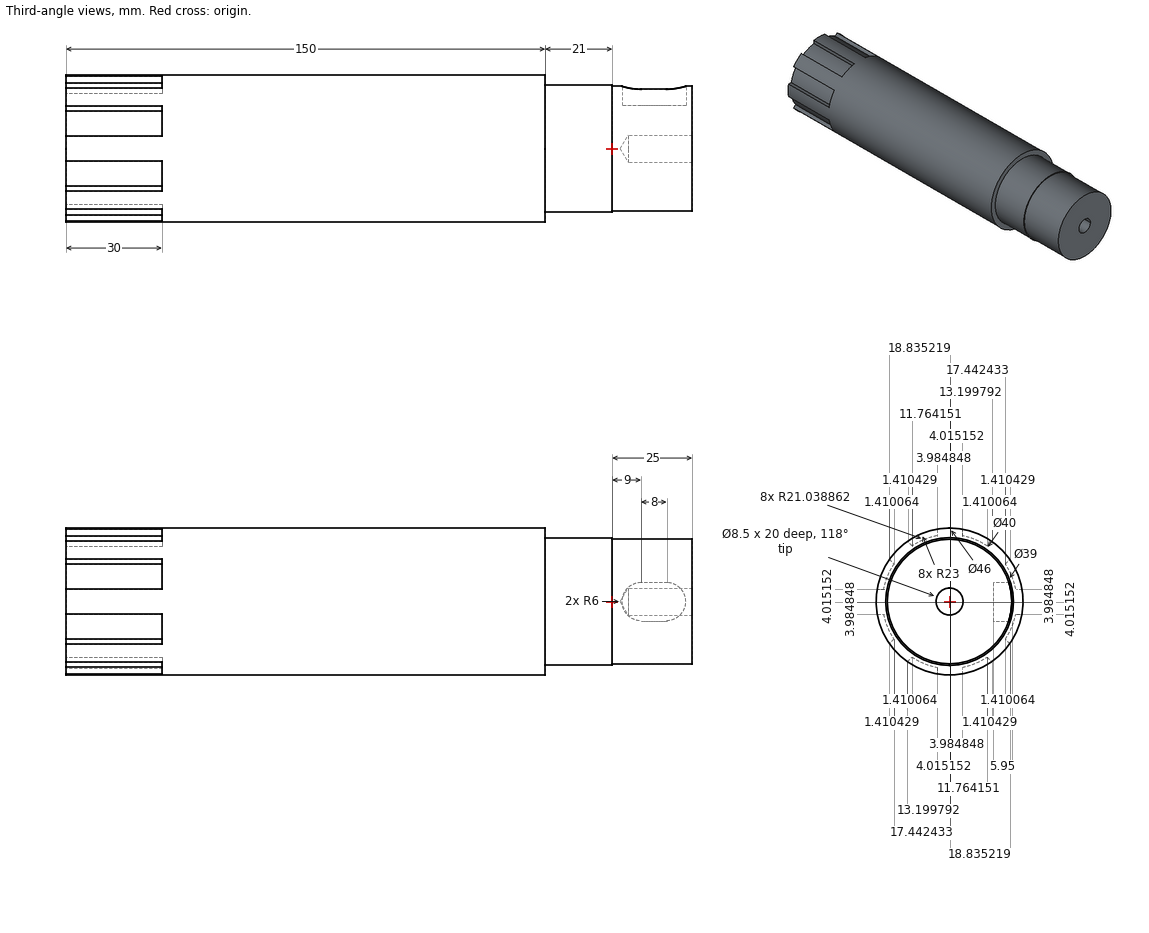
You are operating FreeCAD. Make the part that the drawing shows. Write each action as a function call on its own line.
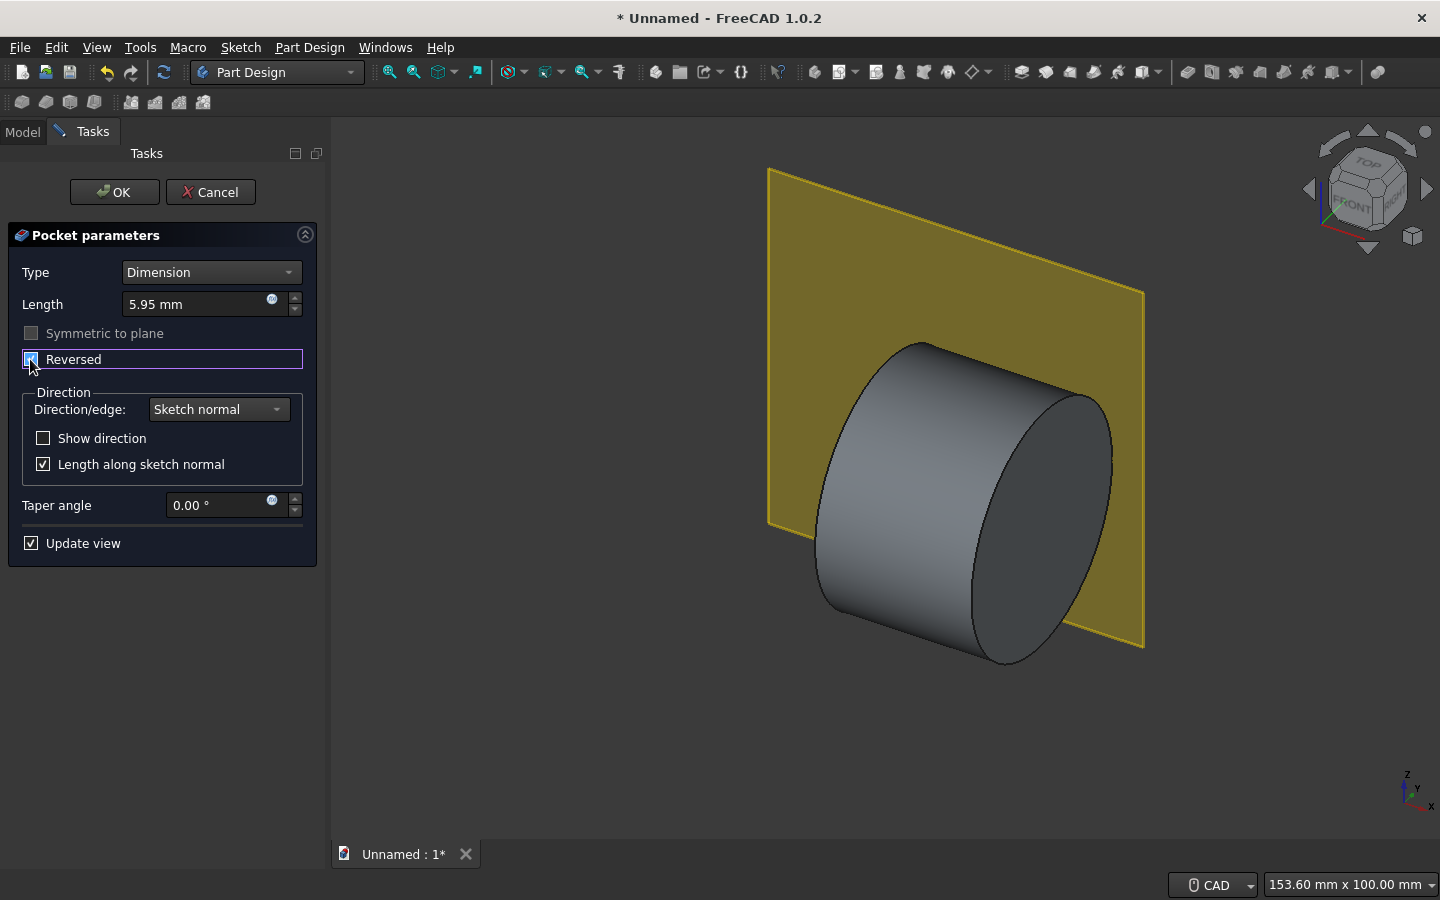
click(115, 192)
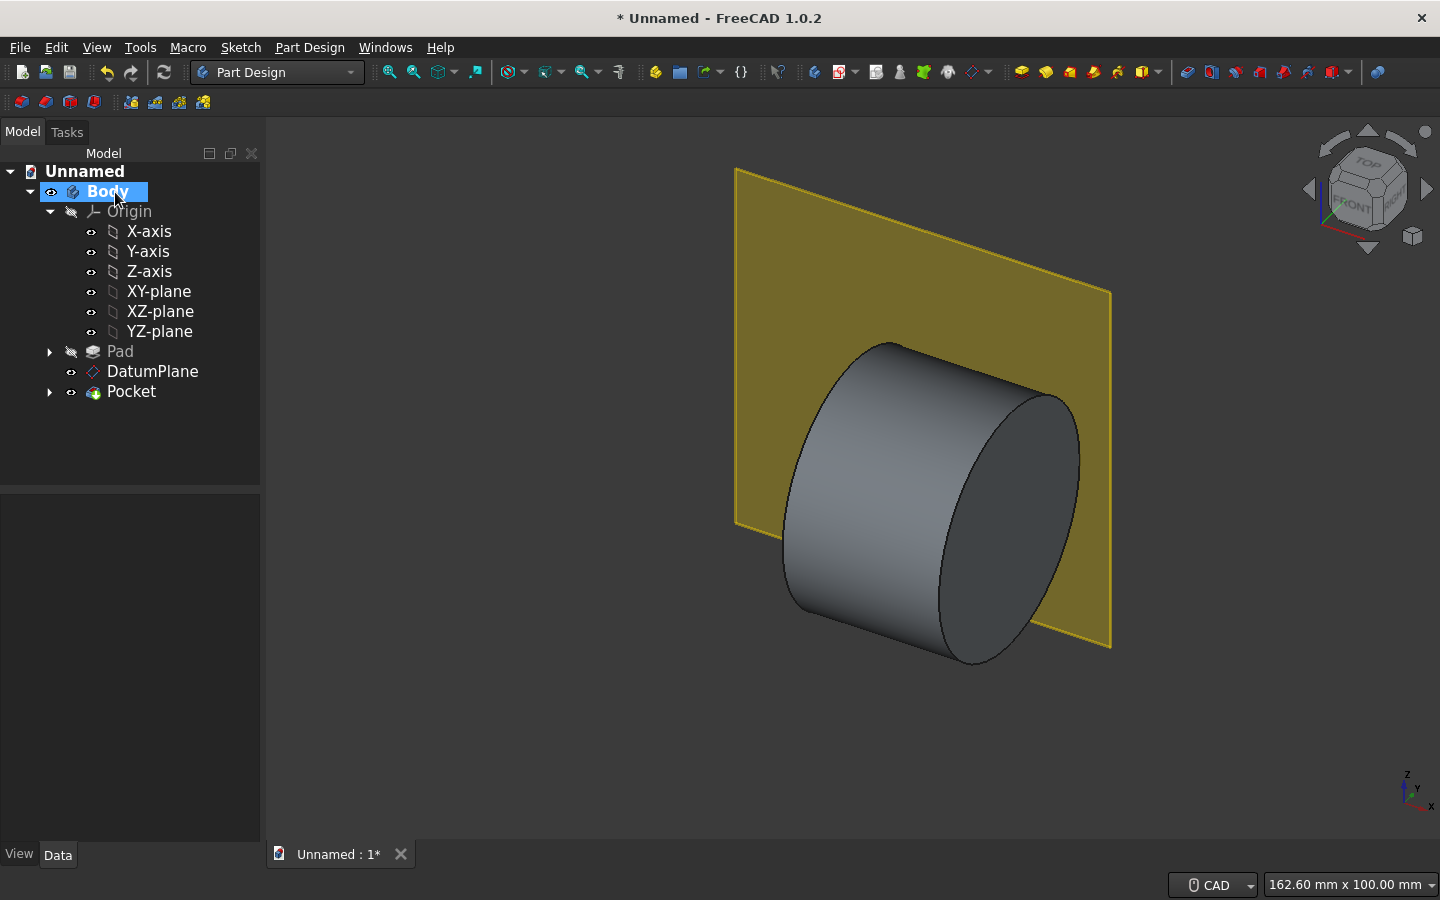
click(116, 372)
key(space)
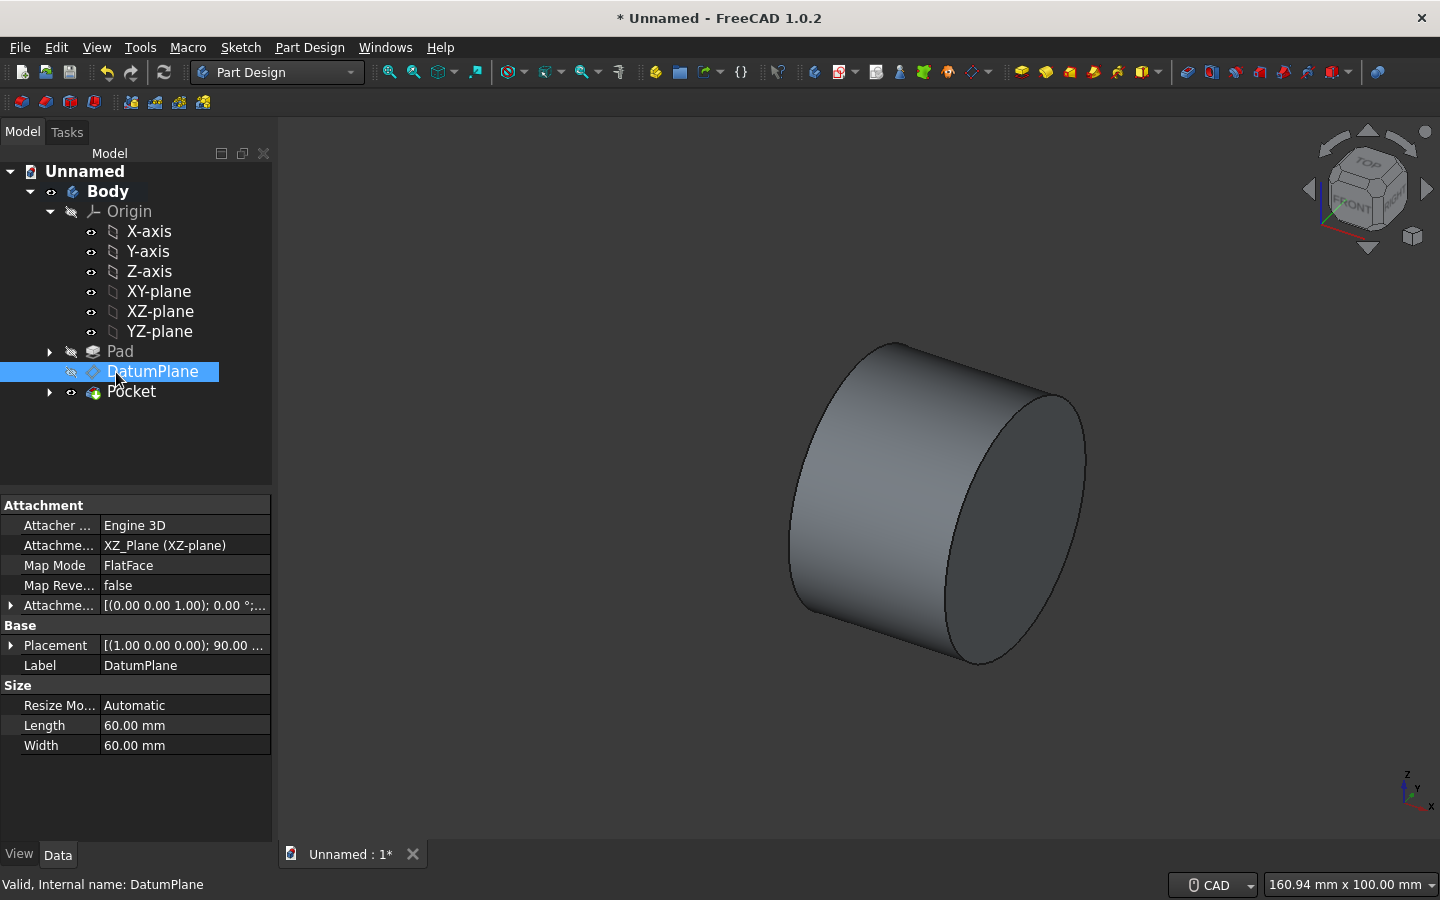
click(318, 799)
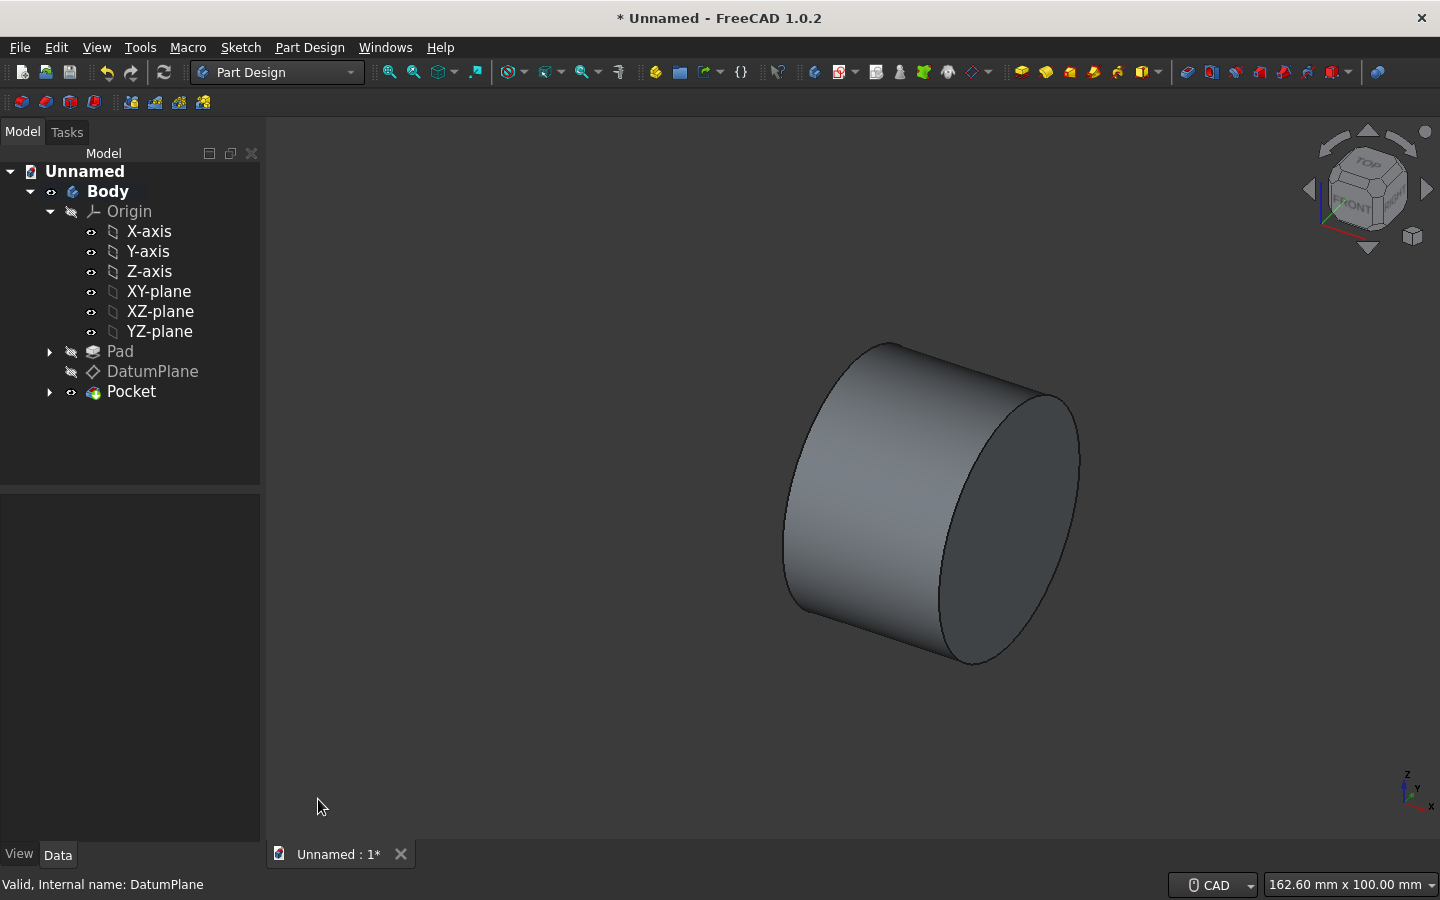
click(840, 72)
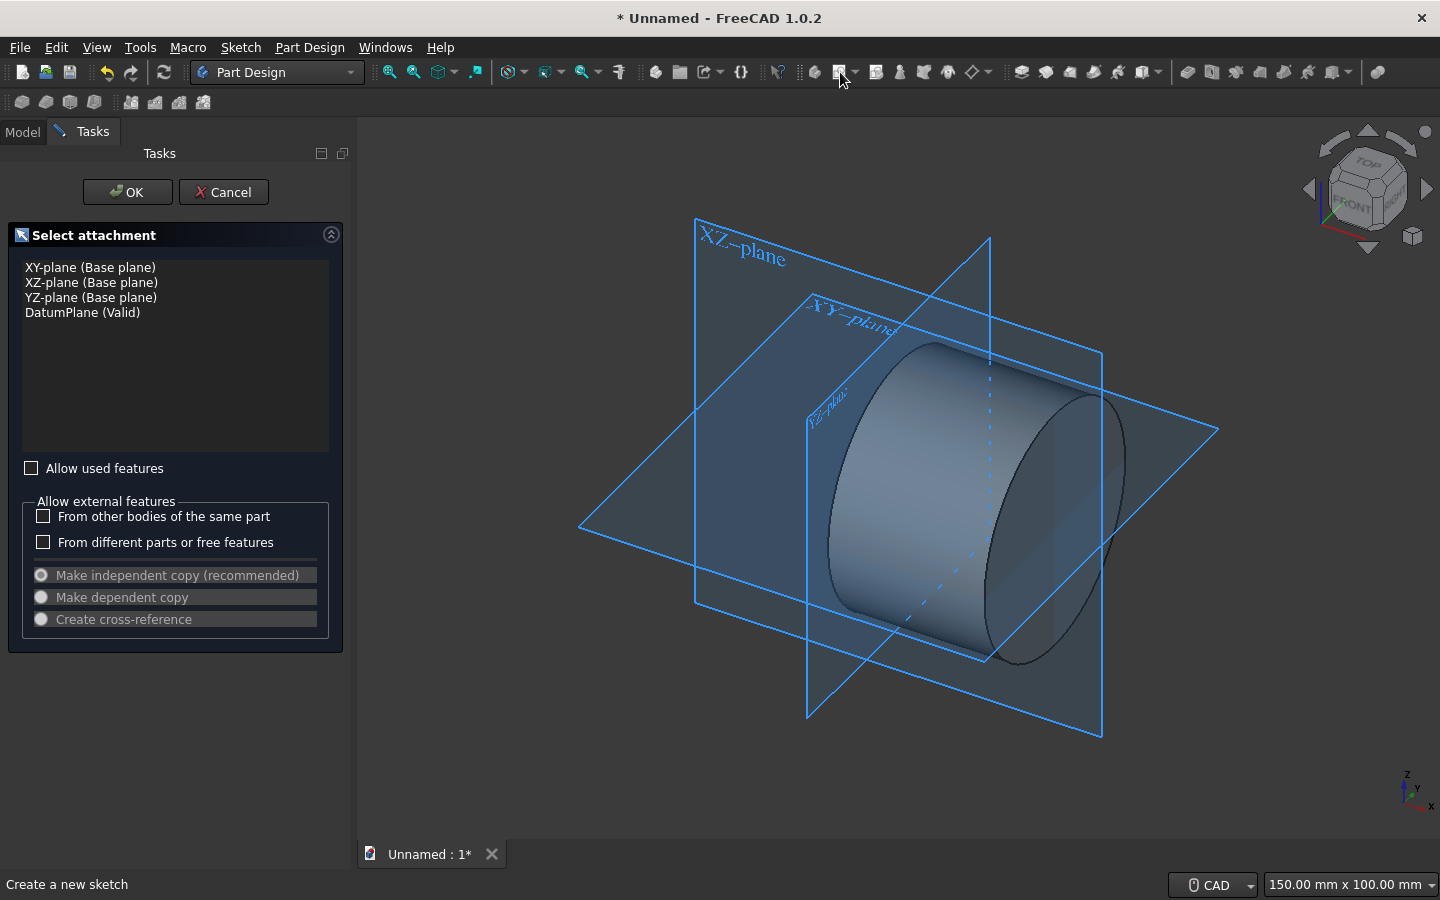
click(82, 298)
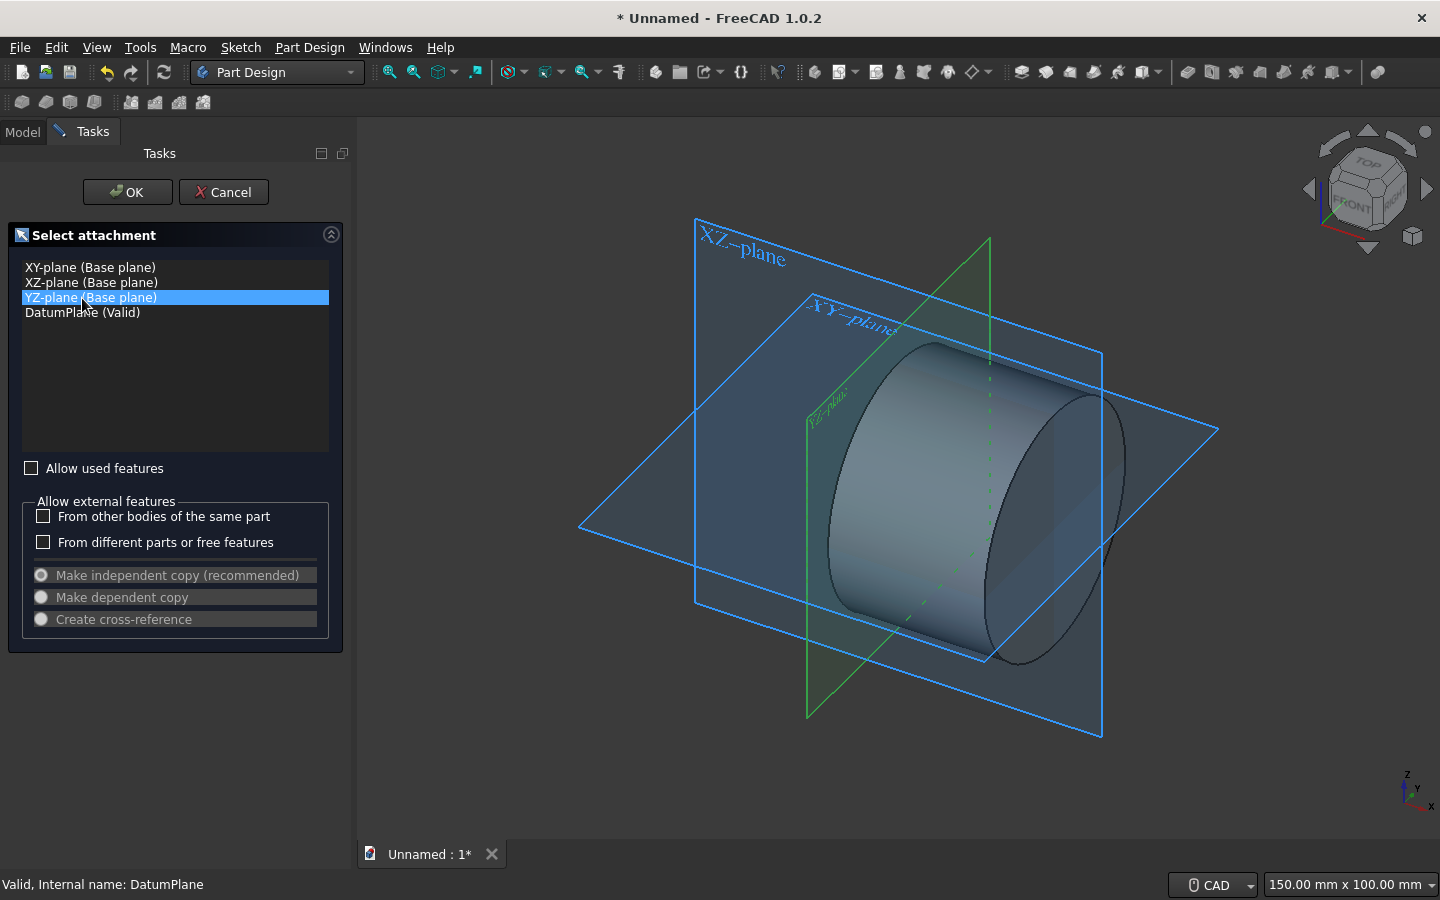
click(128, 192)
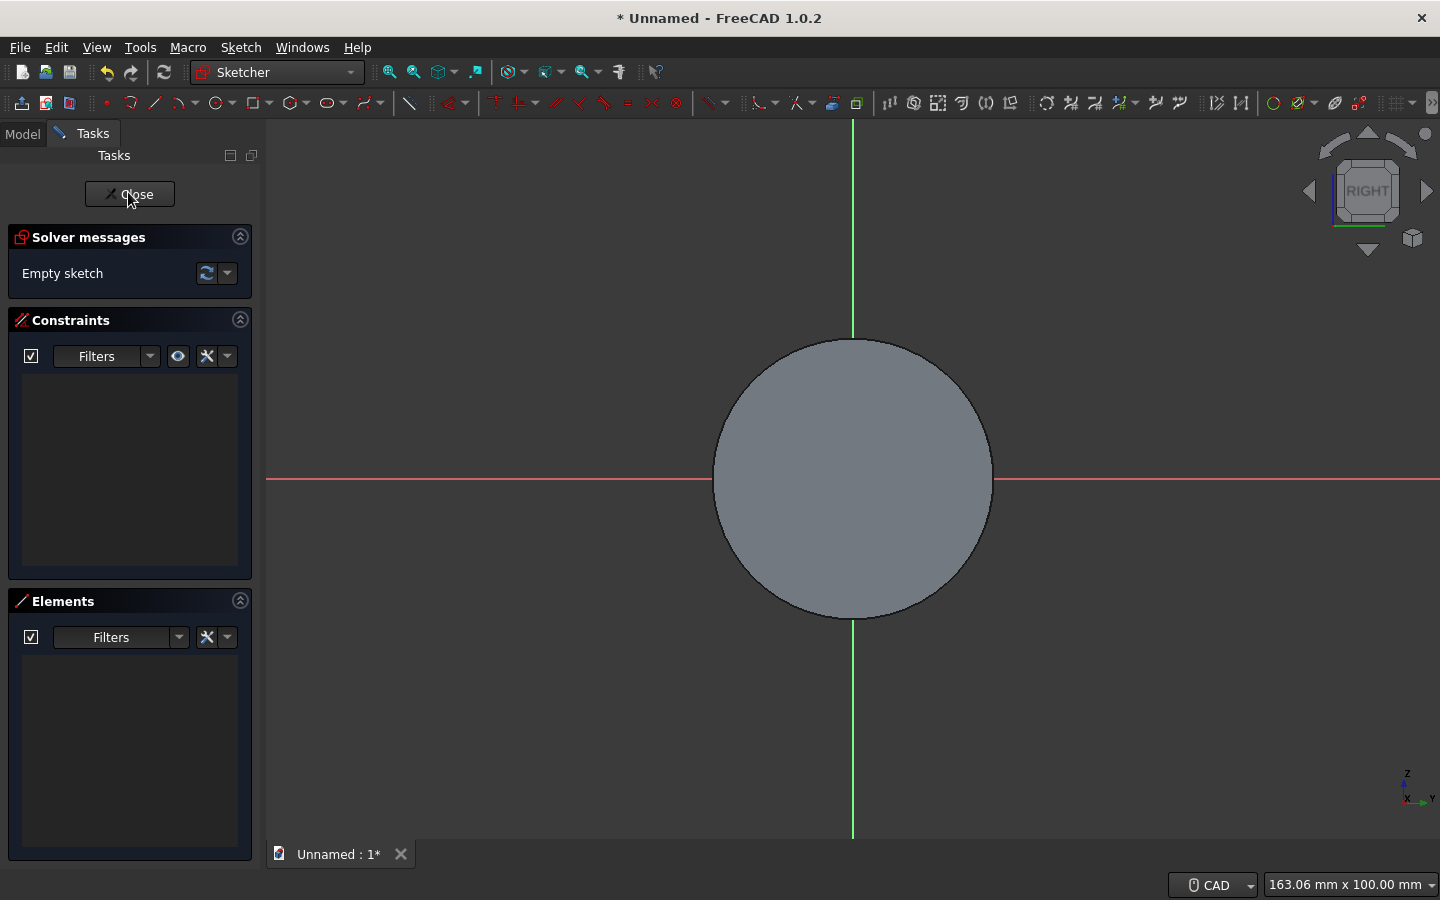
click(70, 104)